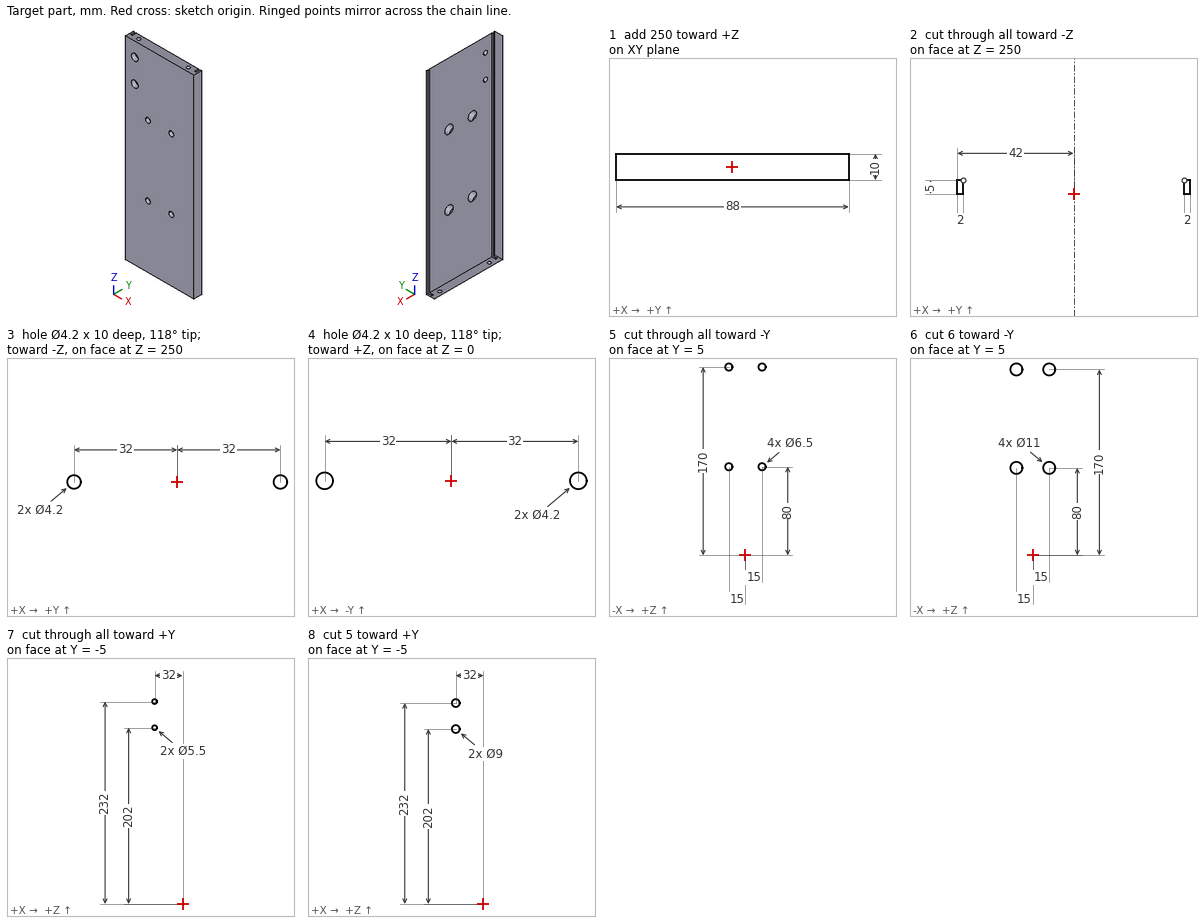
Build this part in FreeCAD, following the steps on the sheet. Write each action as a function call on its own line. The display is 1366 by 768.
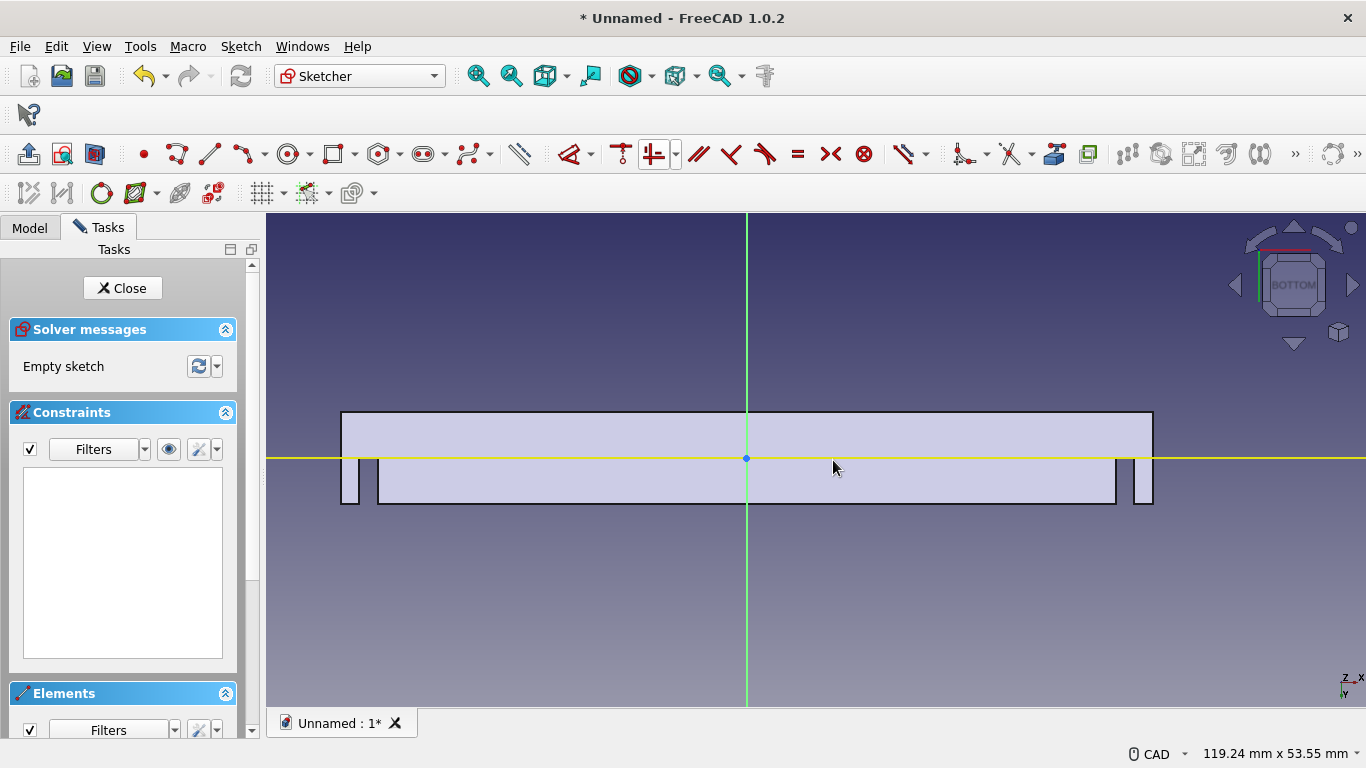
click(288, 154)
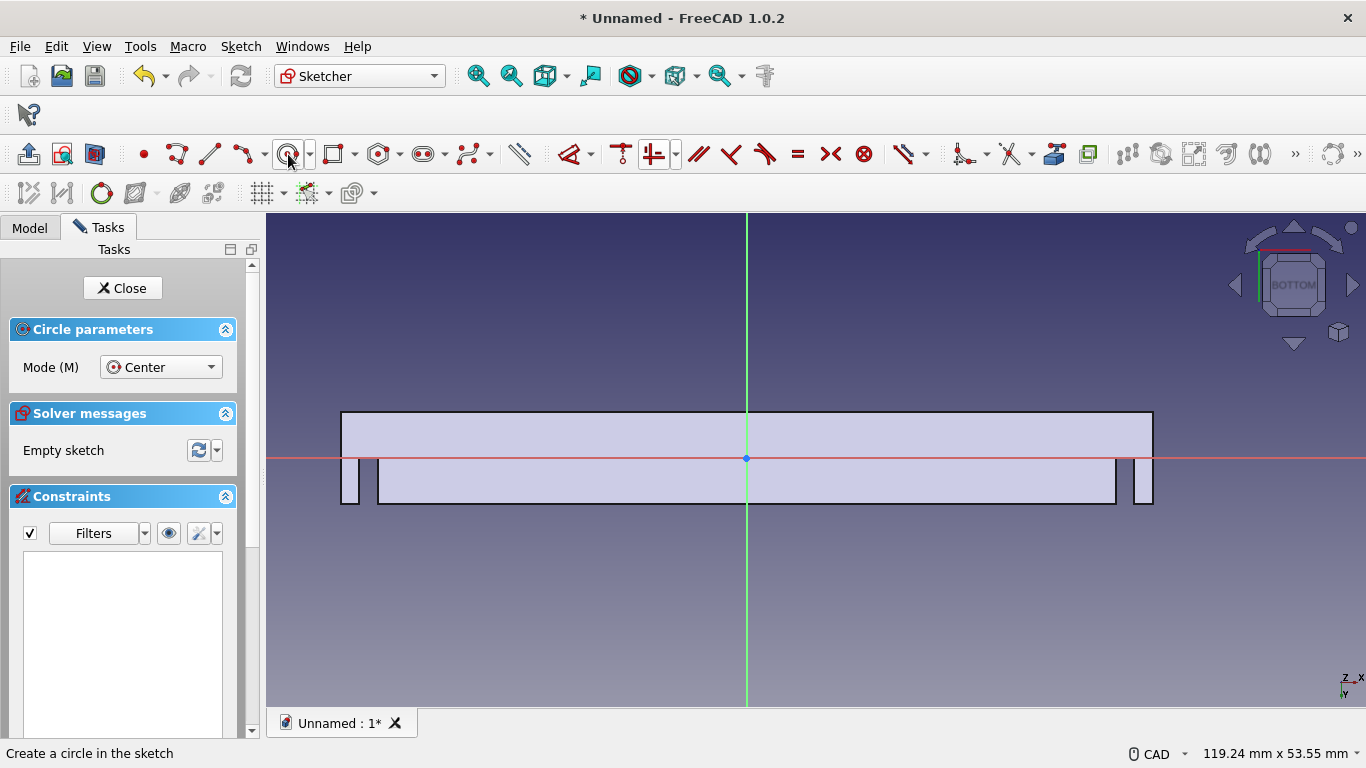
click(1042, 458)
move(1049, 440)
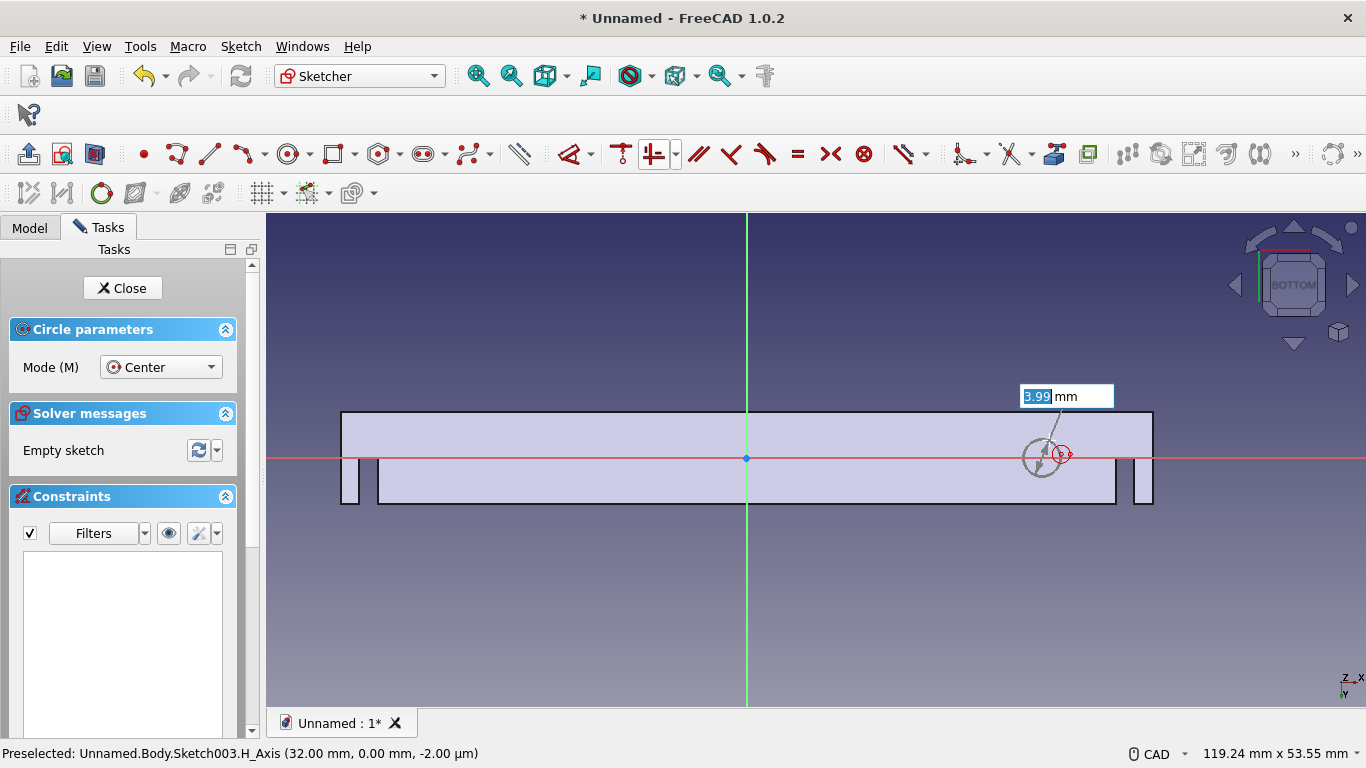
text(4.2)
key(Return)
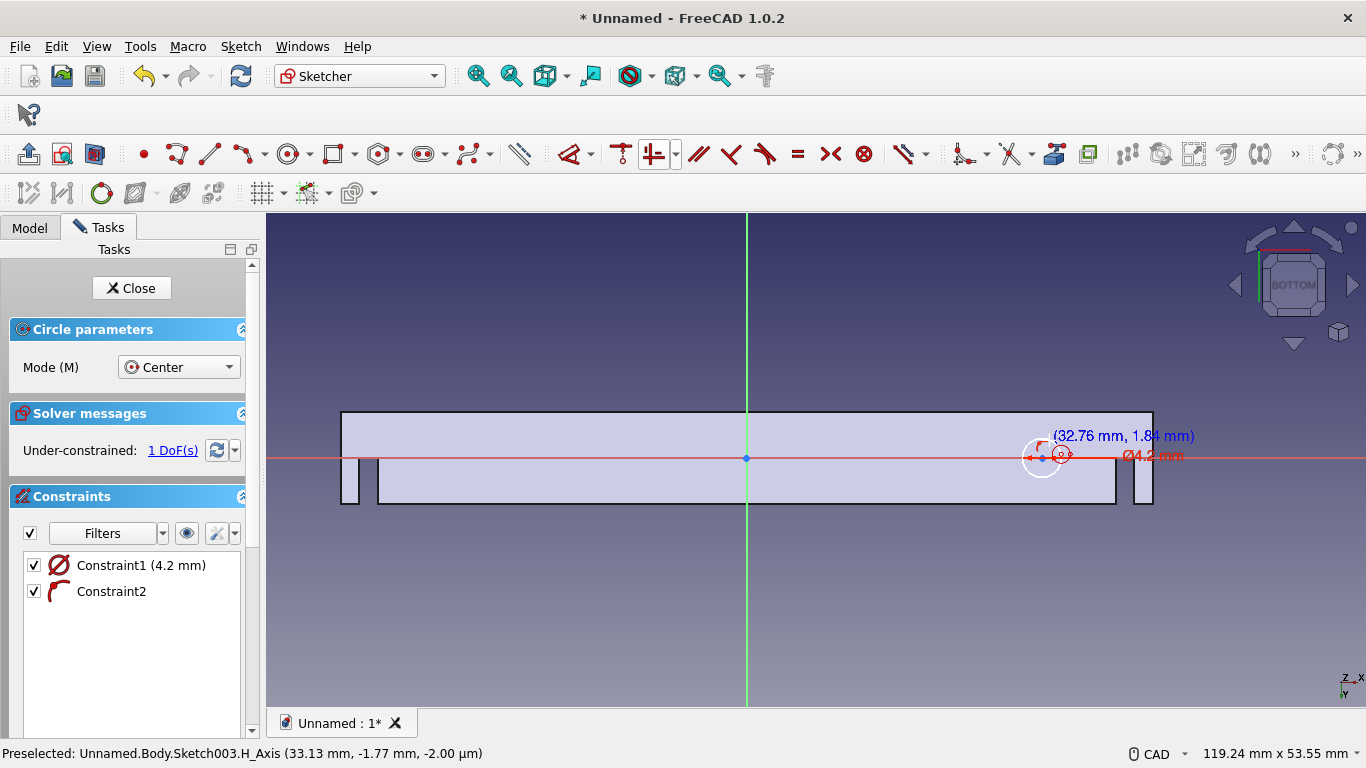
click(452, 458)
move(458, 440)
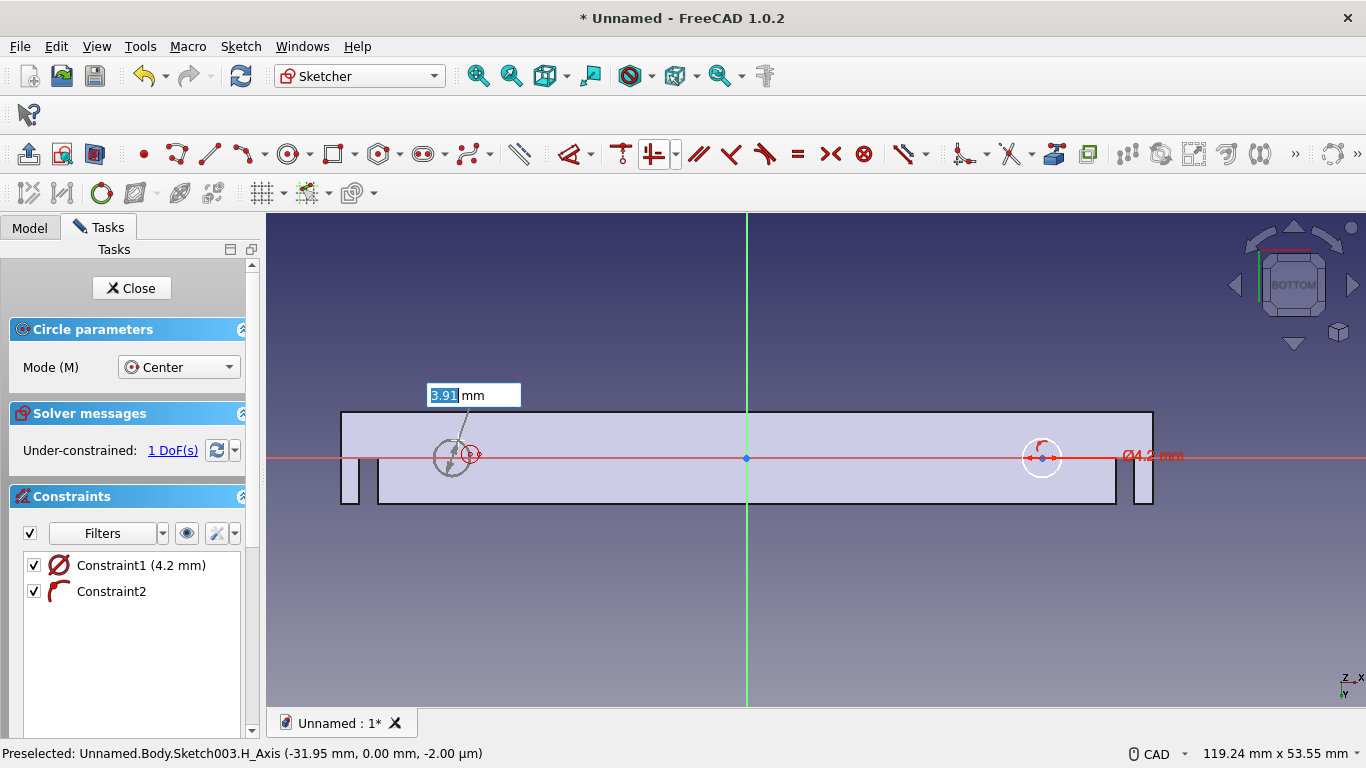
text(4.2)
key(Return)
key(Escape)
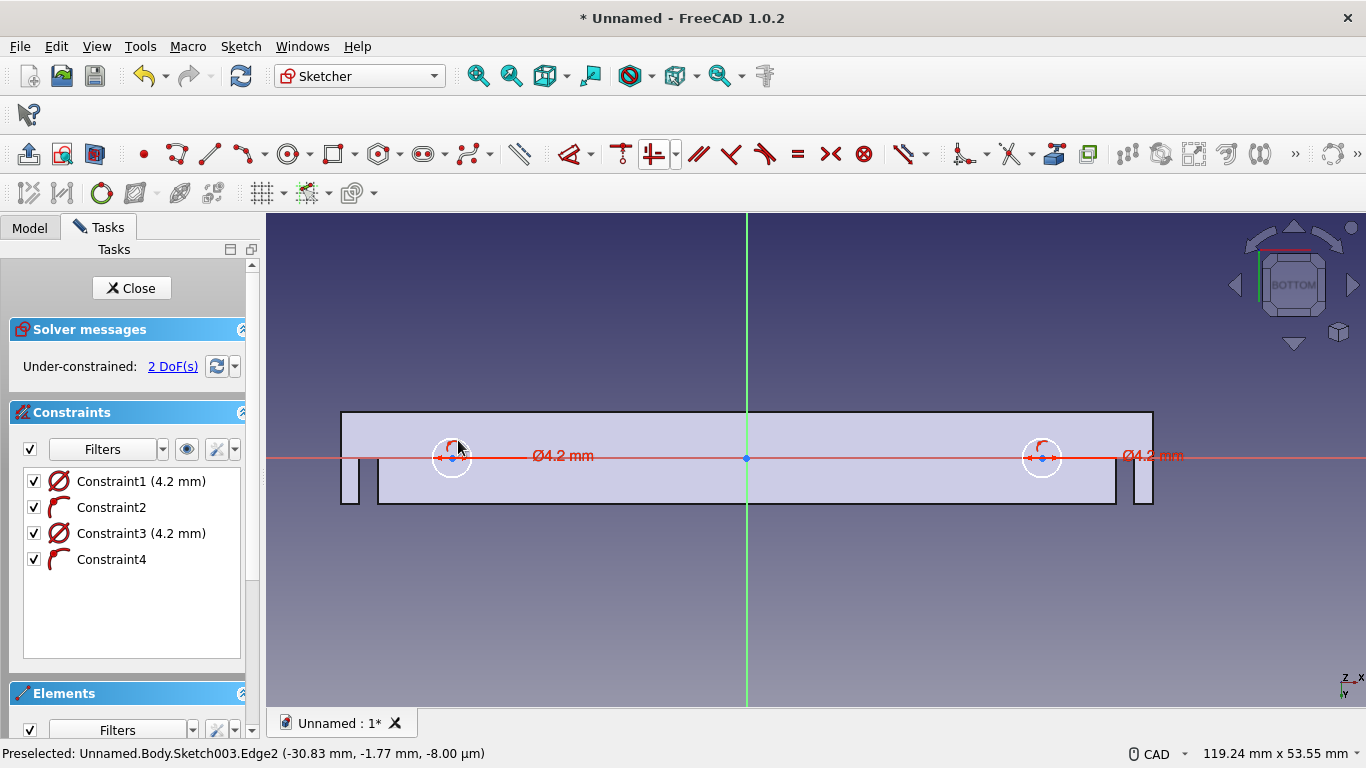
click(568, 154)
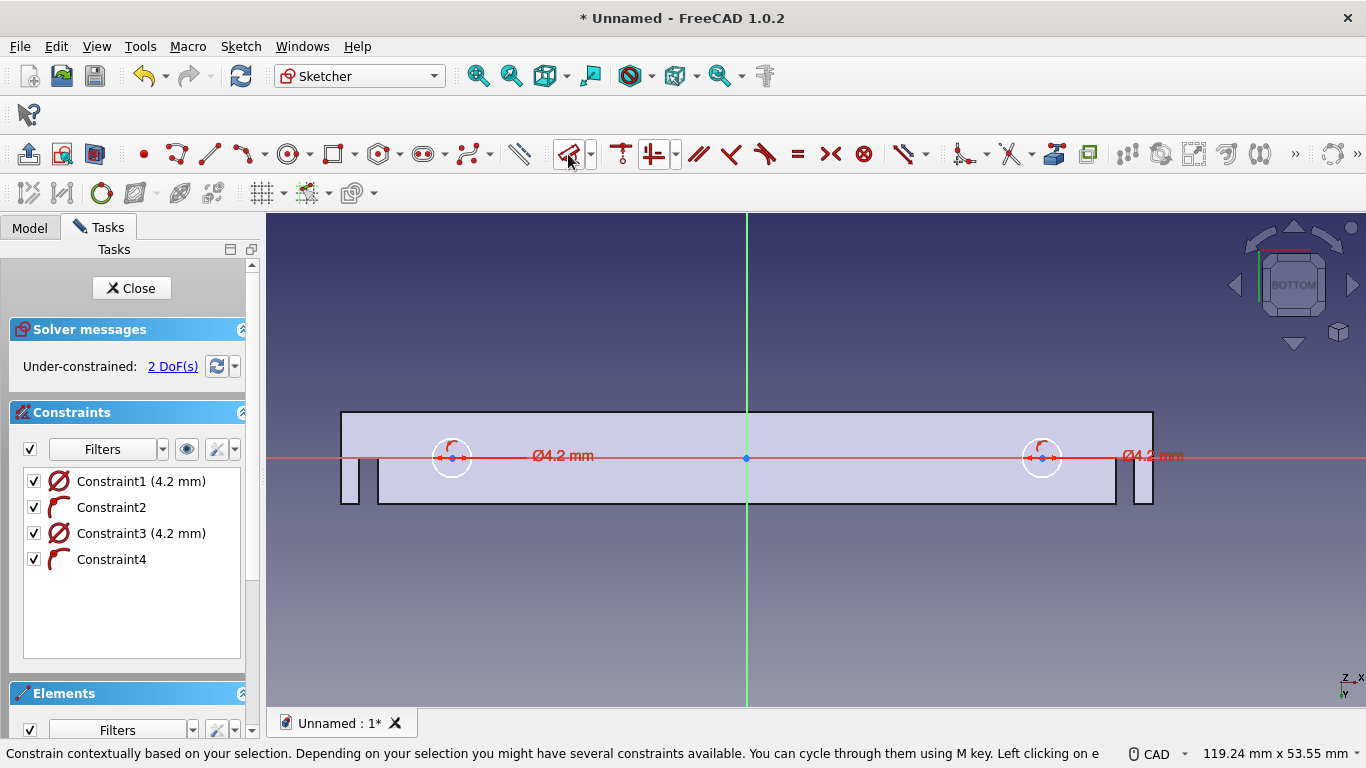
click(1042, 458)
click(894, 492)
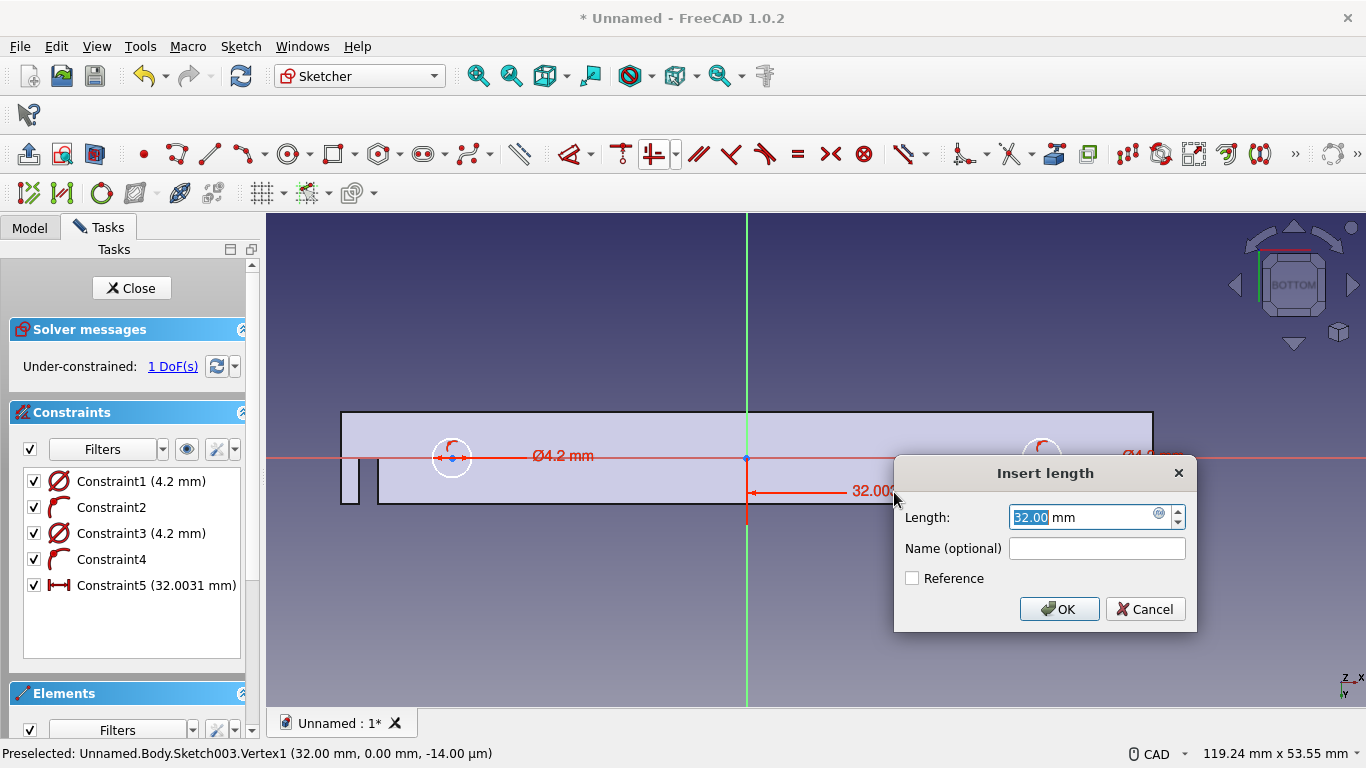
text(32)
key(Return)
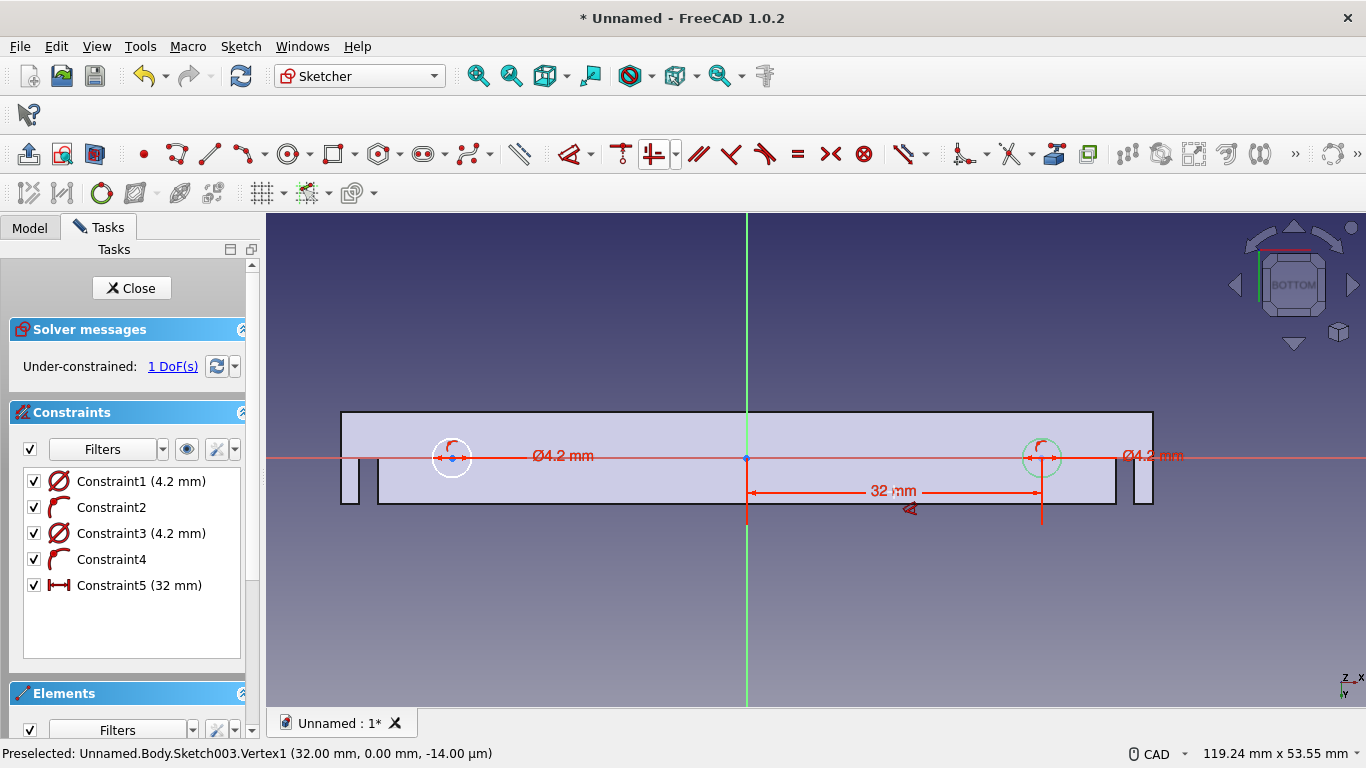
click(452, 458)
click(599, 492)